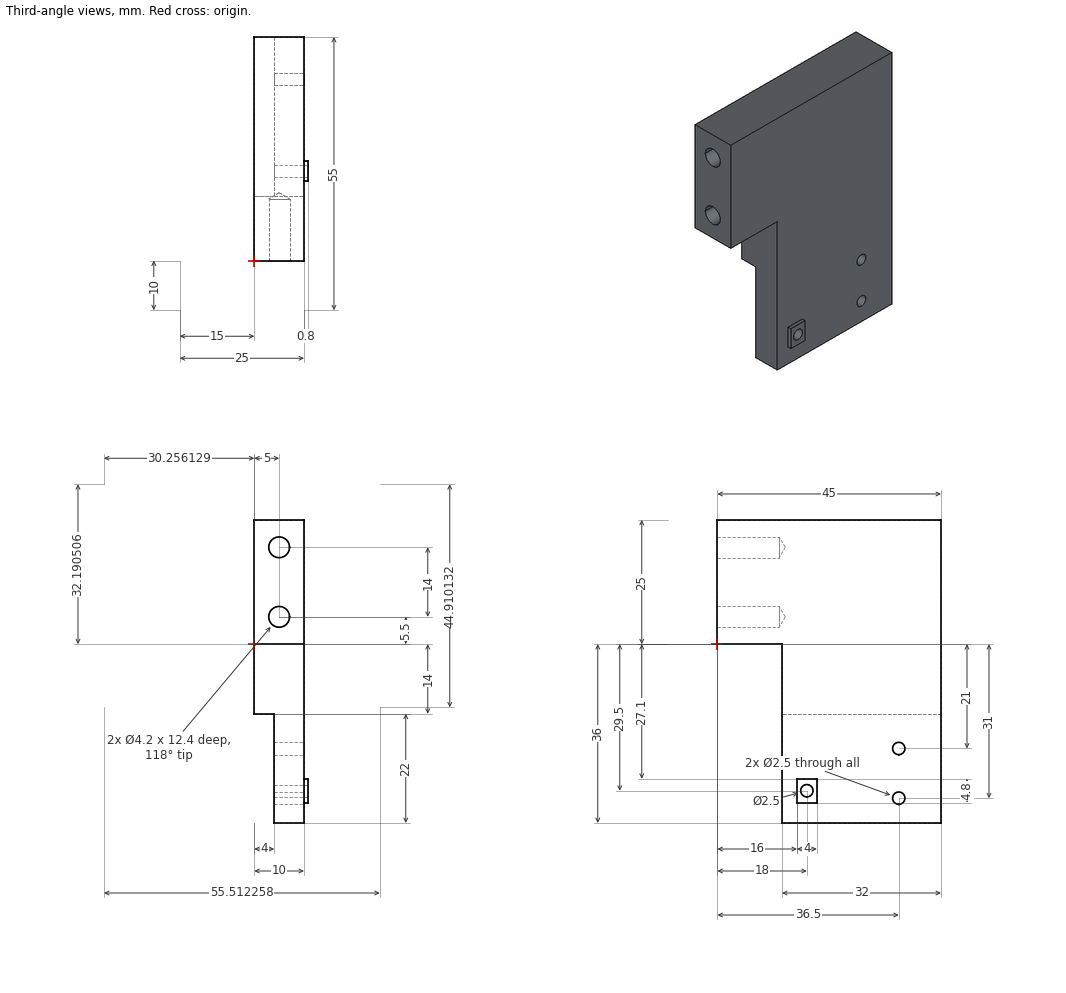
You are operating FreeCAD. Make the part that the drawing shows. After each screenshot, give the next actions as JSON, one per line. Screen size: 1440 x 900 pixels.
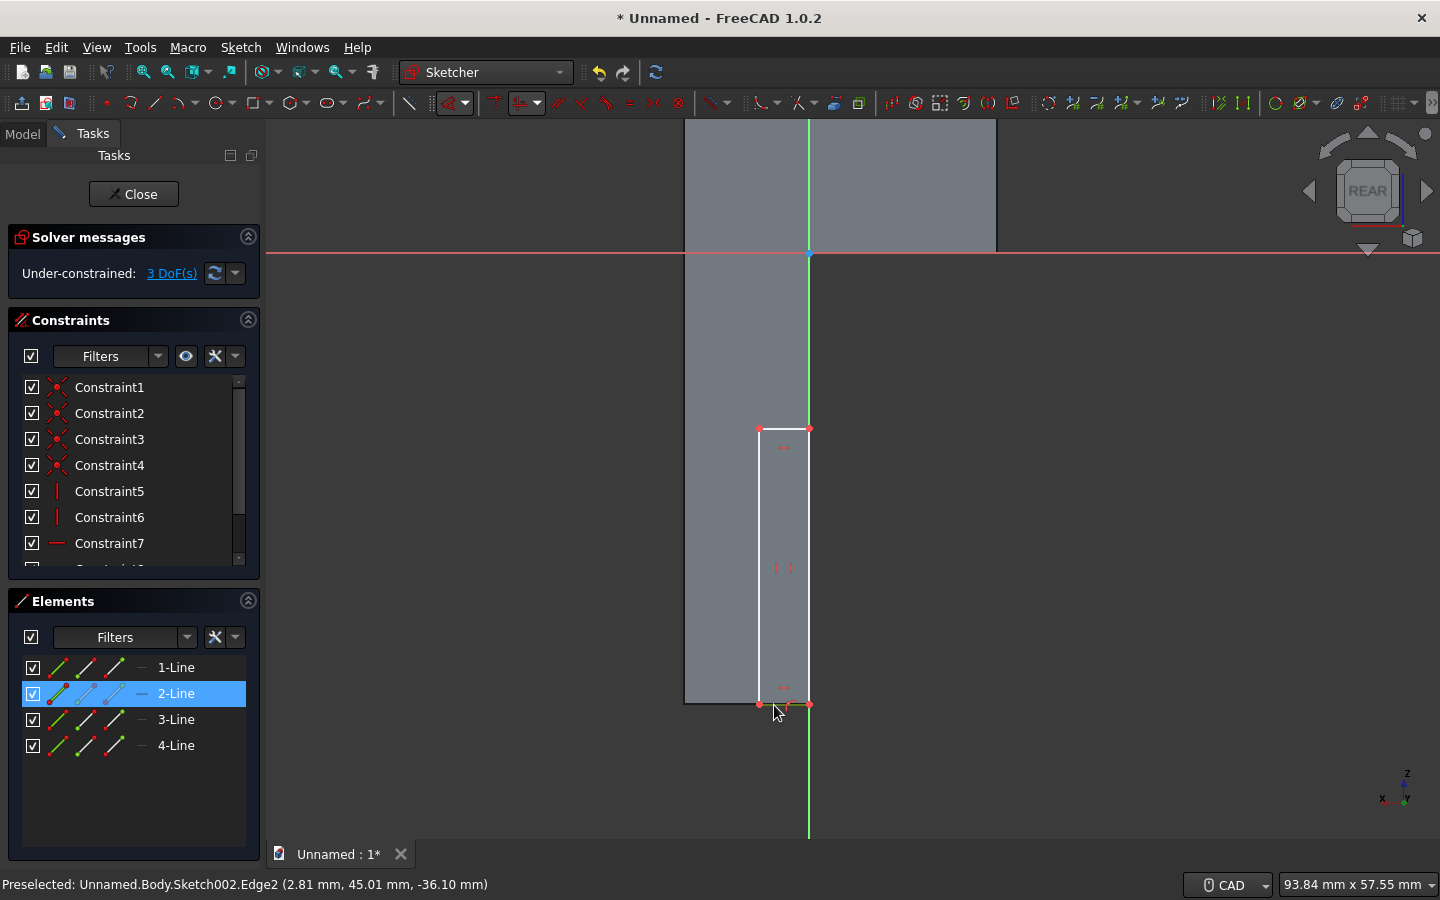
{"action": "key", "text": "l"}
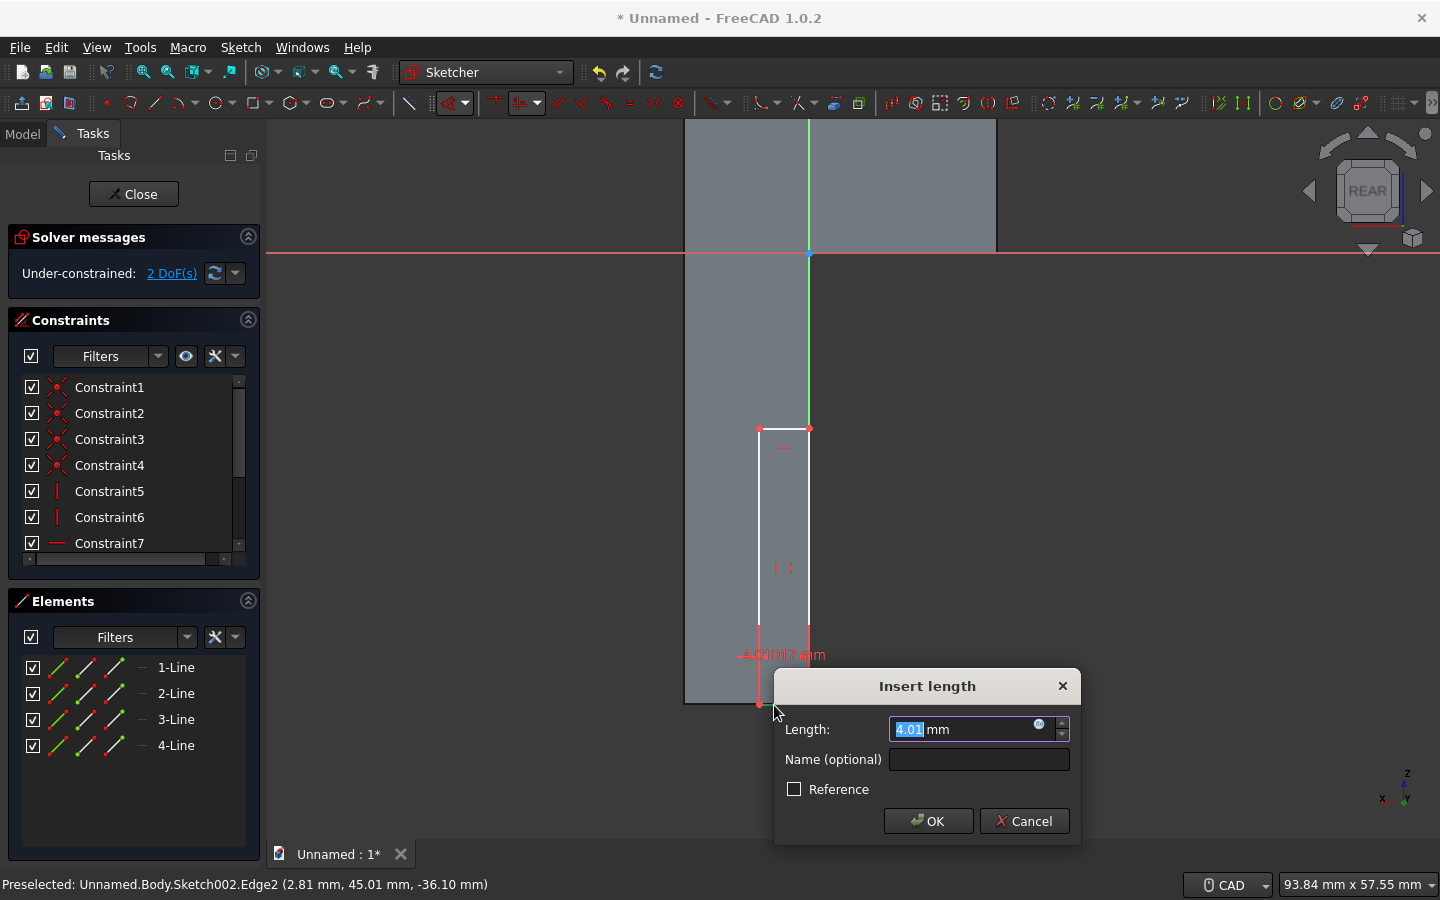
{"action": "type", "text": "4"}
{"action": "key", "text": "Return"}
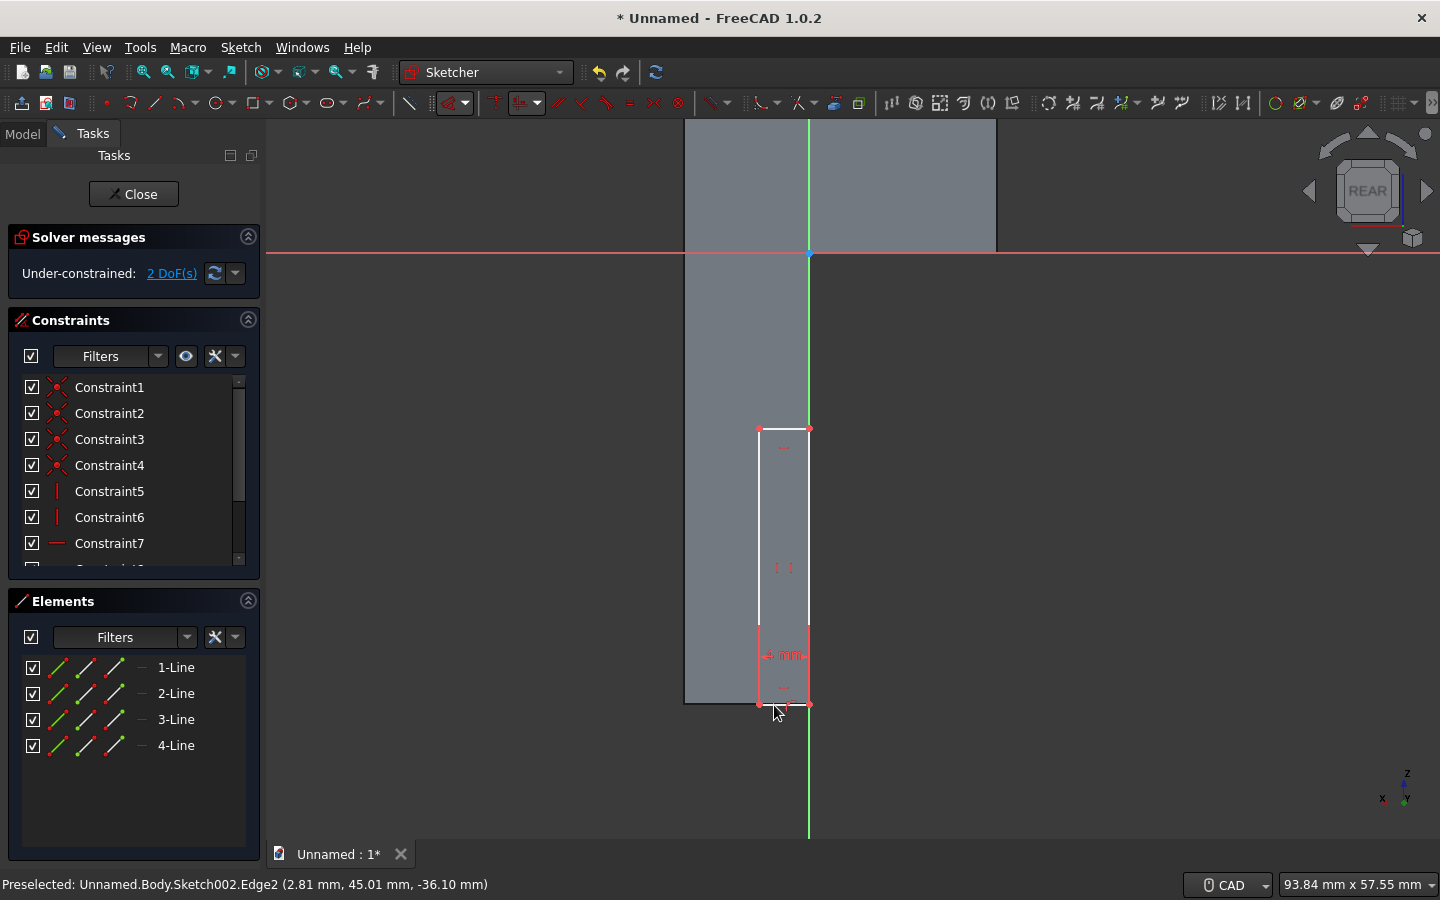
{"action": "left_click", "coordinate": [759, 512]}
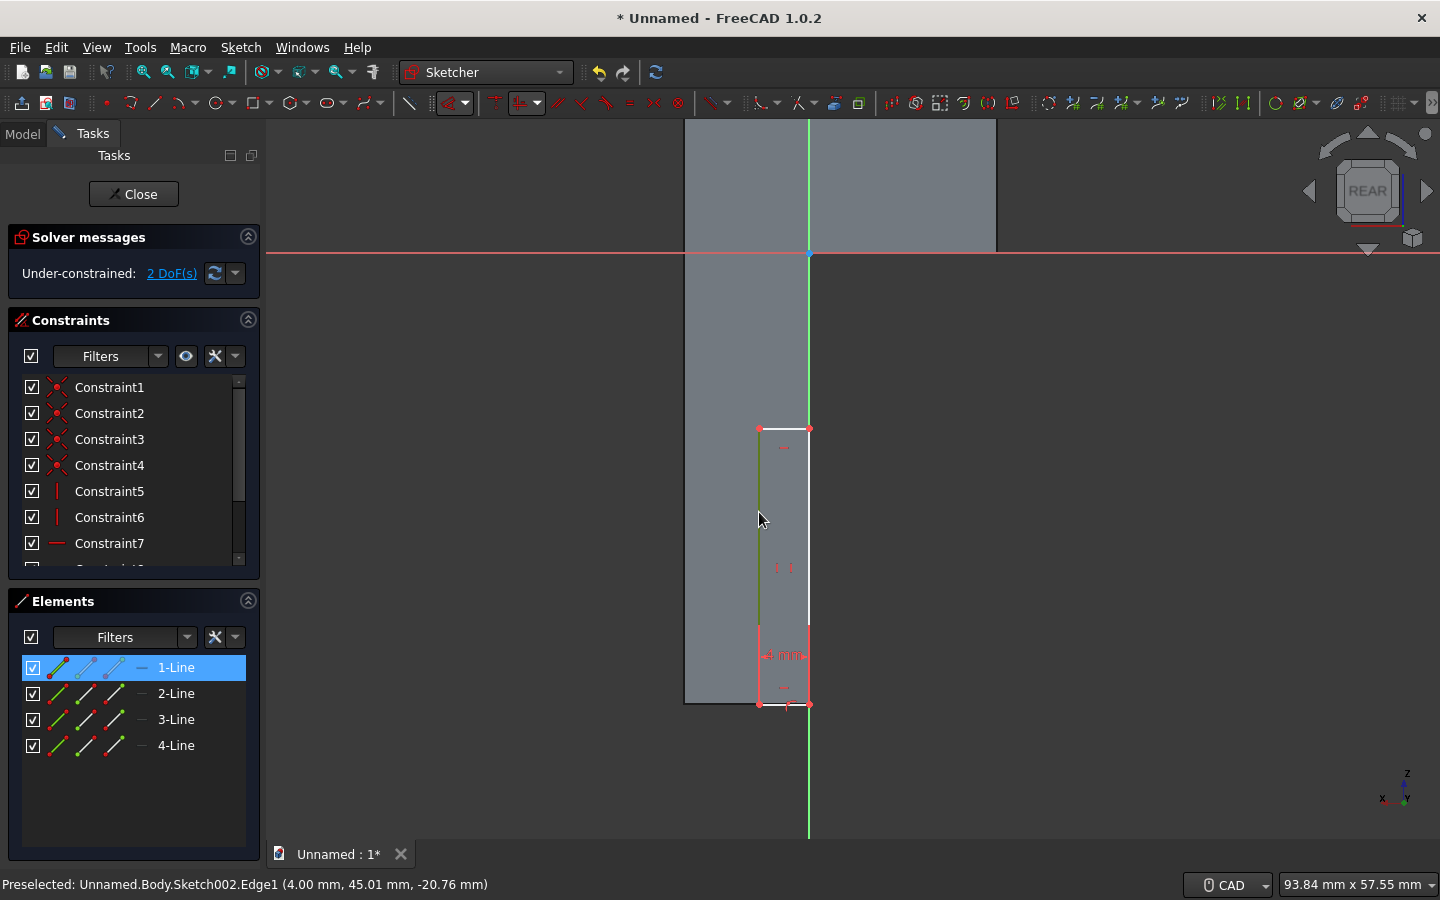
{"action": "key", "text": "i"}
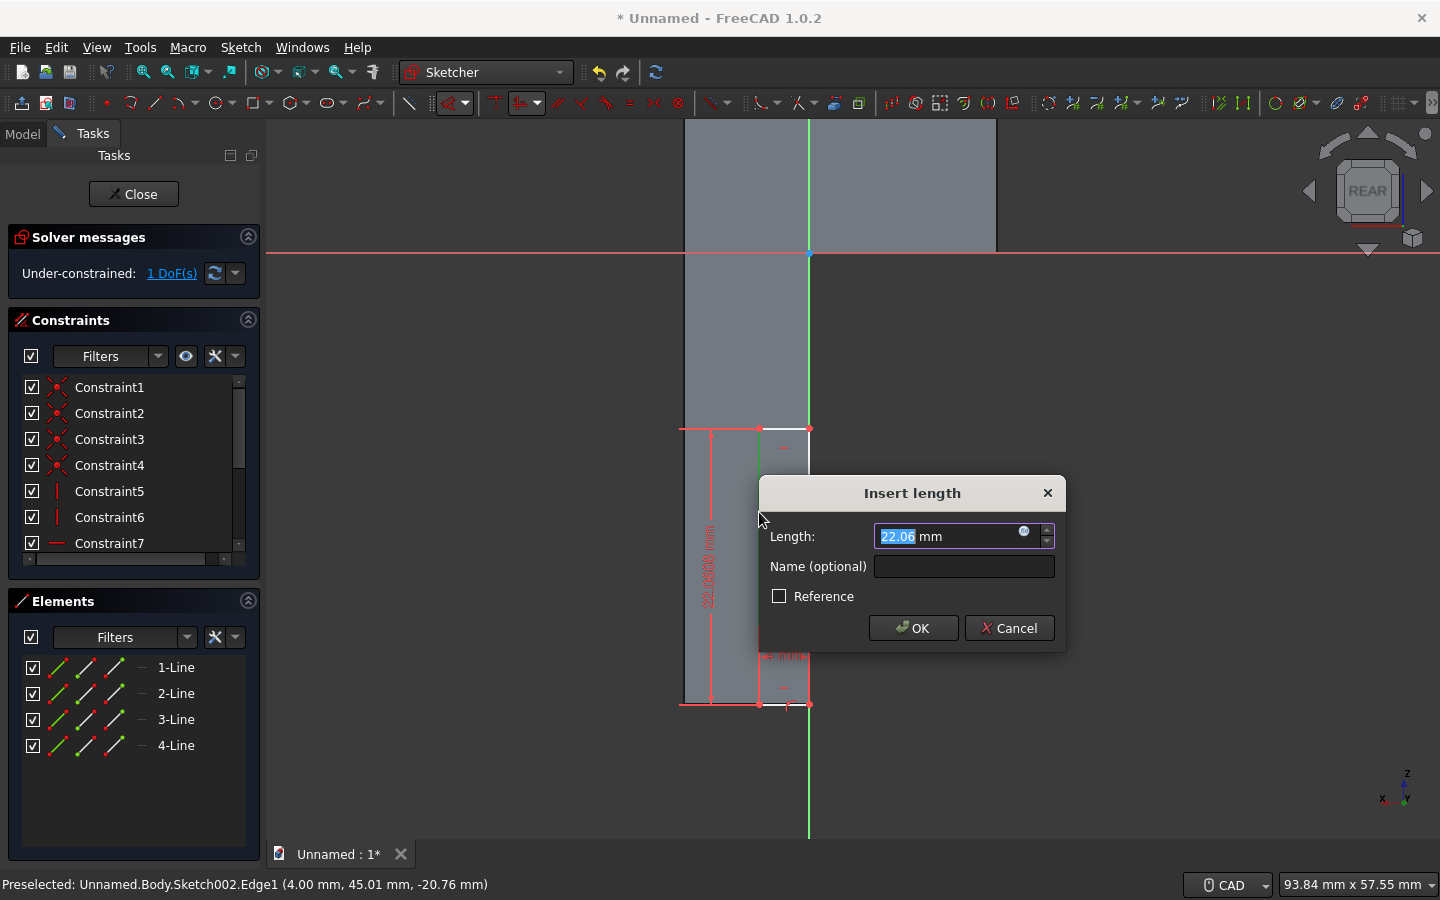
{"action": "type", "text": "22"}
{"action": "key", "text": "Return"}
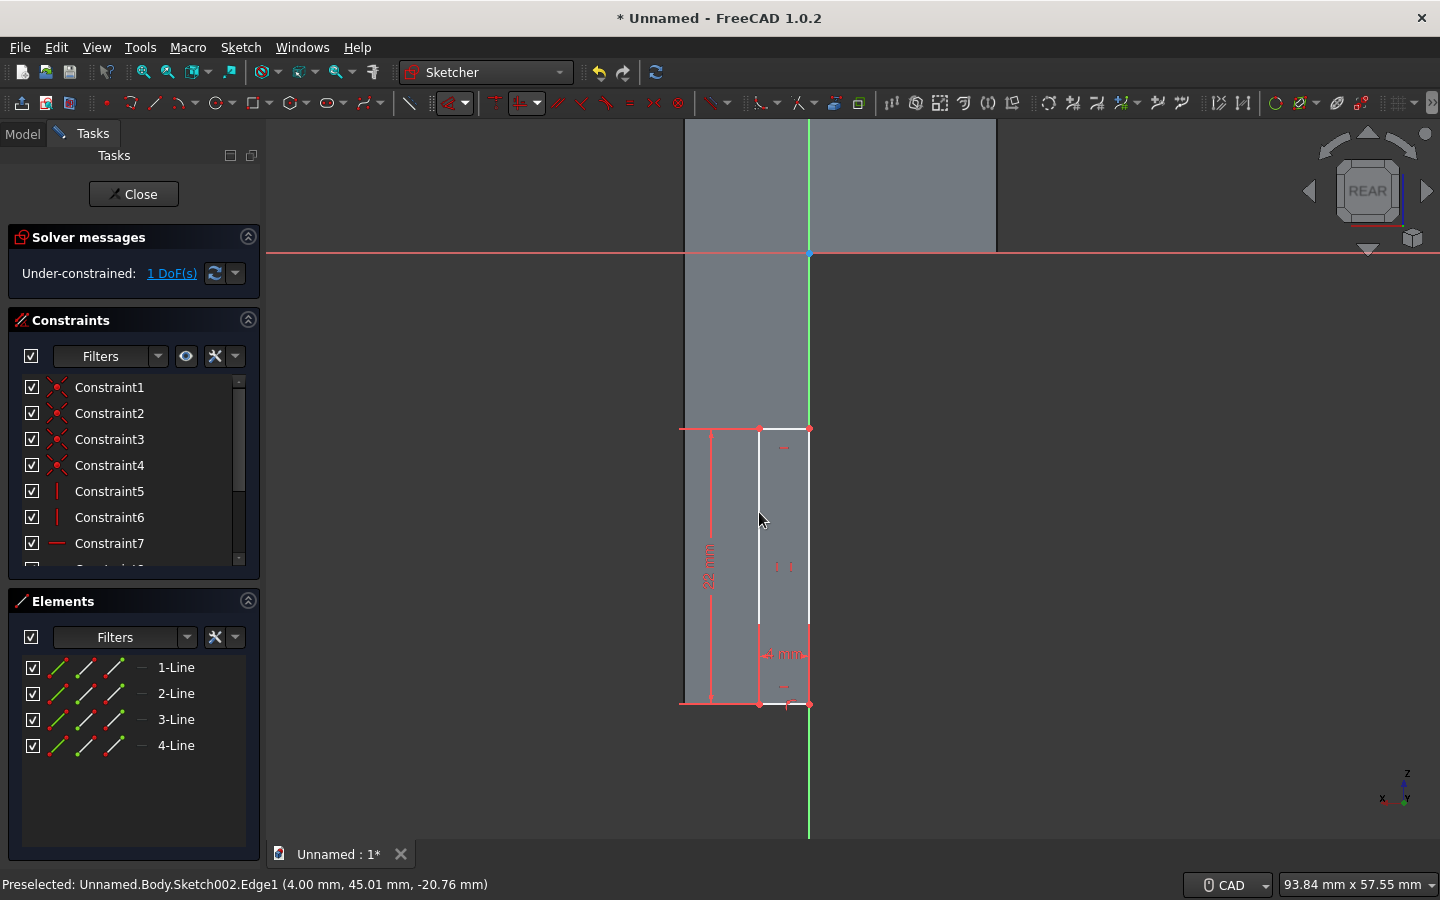
{"action": "left_click", "coordinate": [759, 429]}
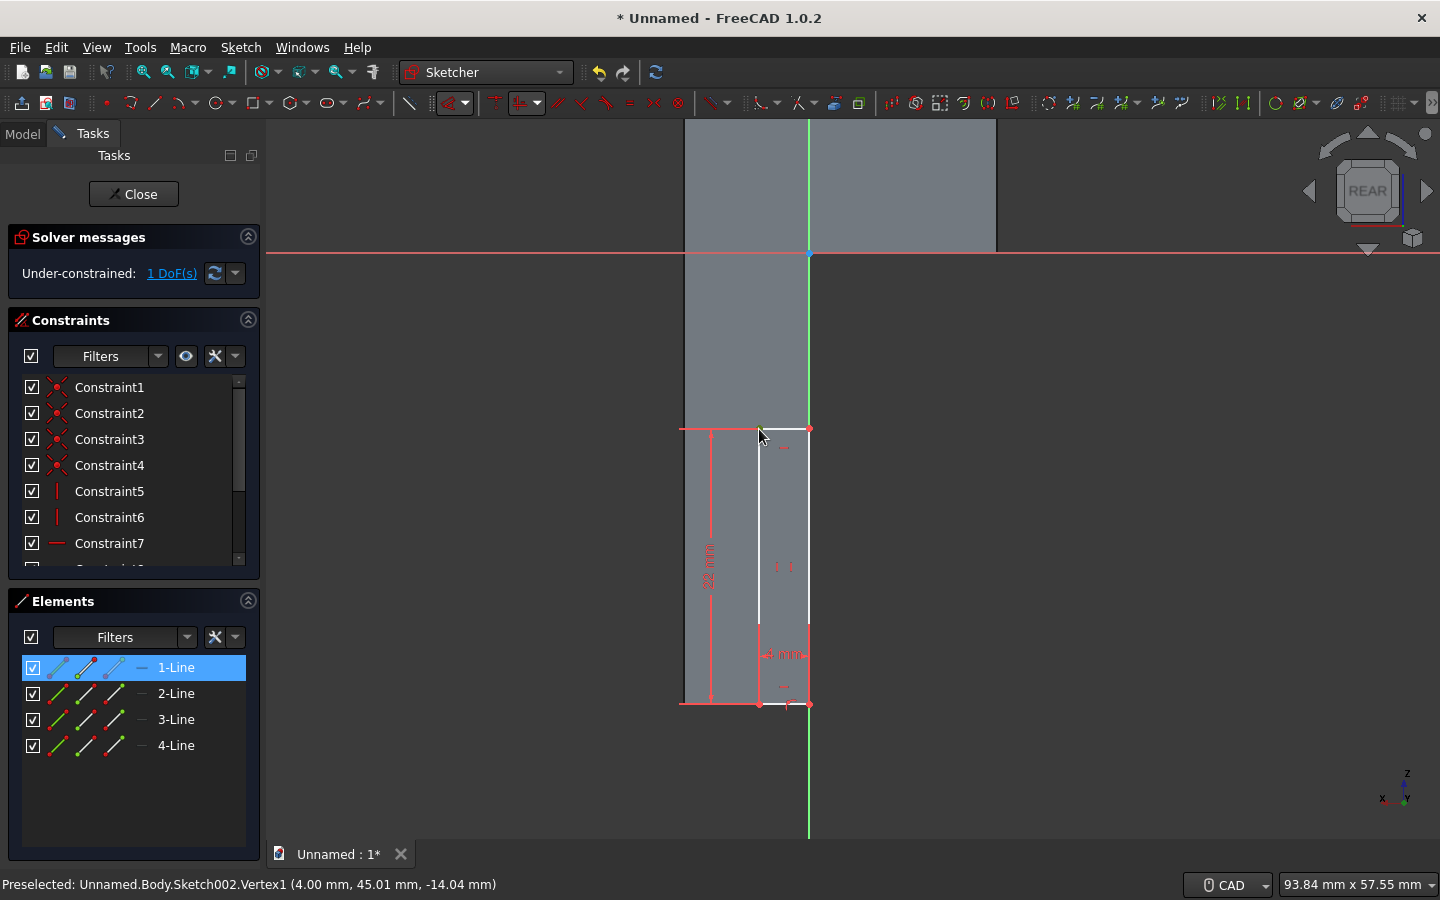
{"action": "key", "text": "i"}